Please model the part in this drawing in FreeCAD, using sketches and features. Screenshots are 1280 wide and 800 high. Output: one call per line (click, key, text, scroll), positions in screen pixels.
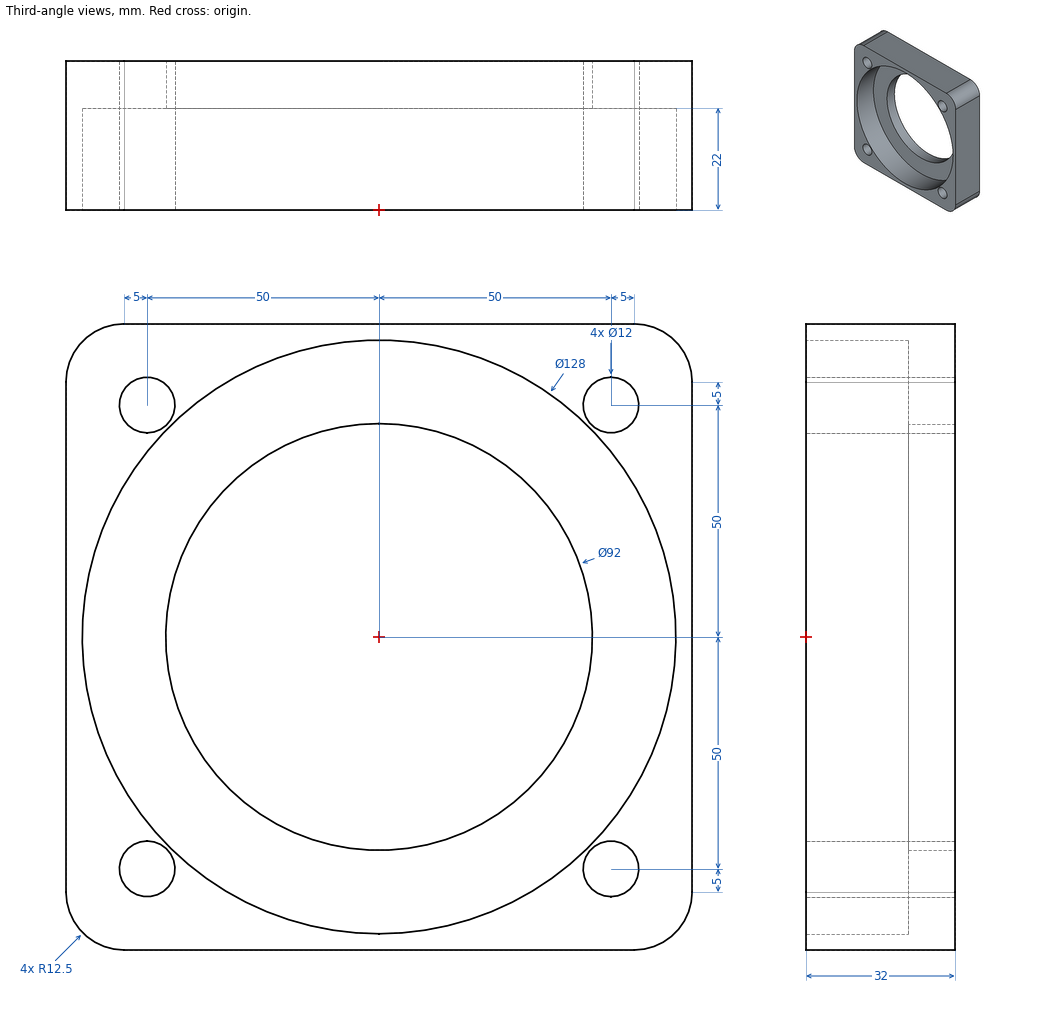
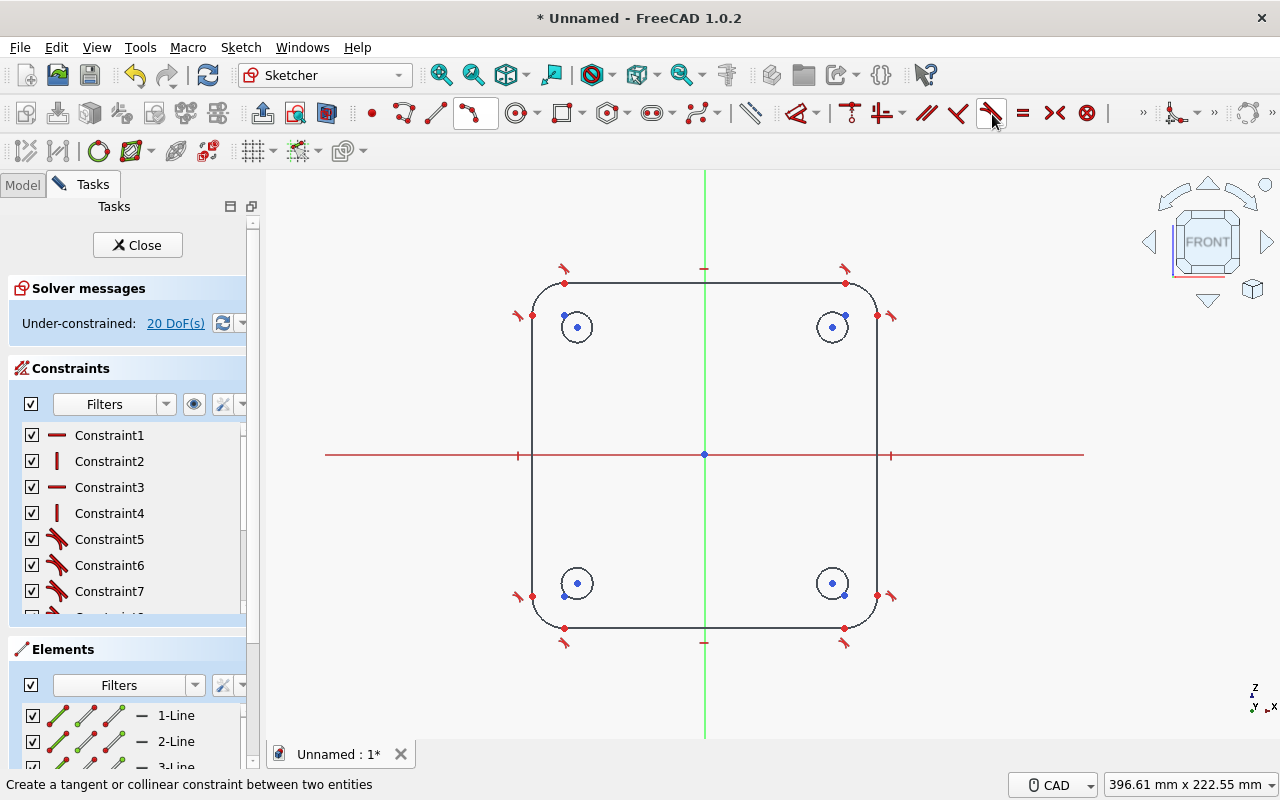
click(536, 611)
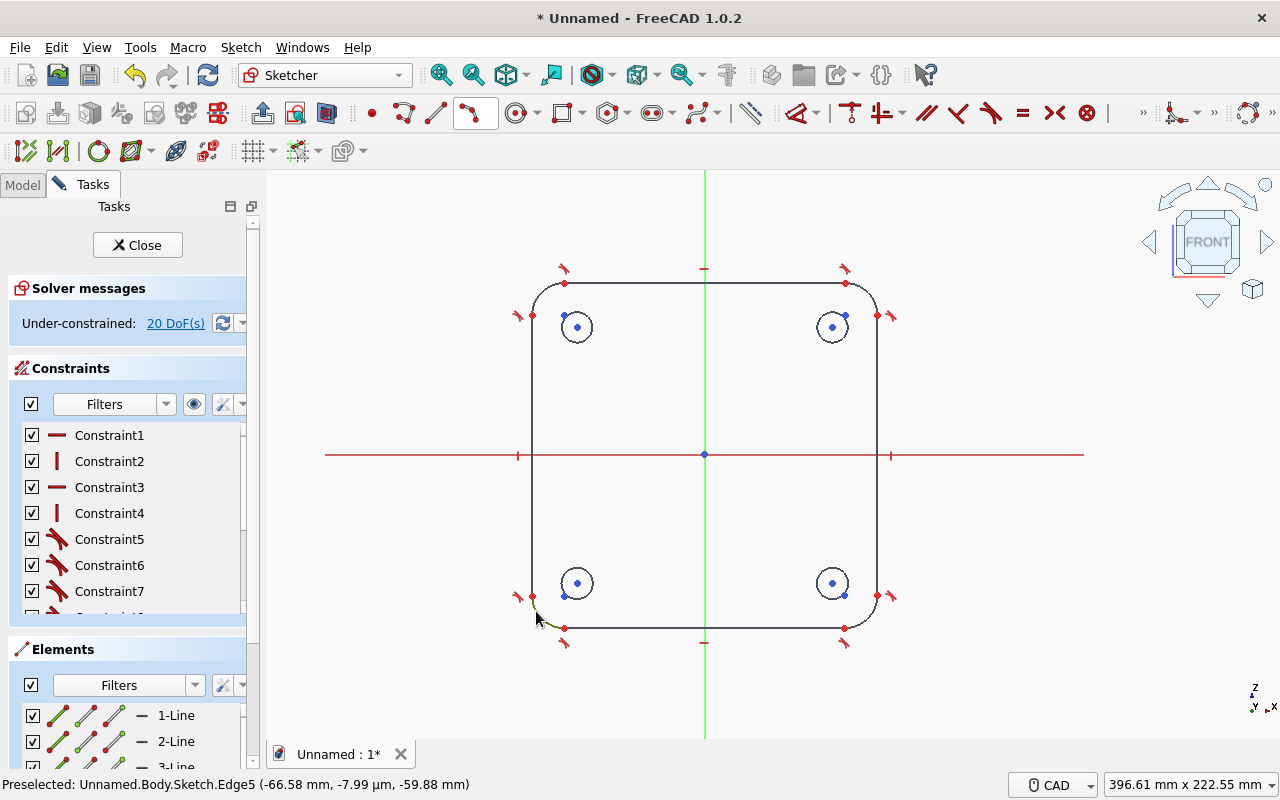
click(550, 287)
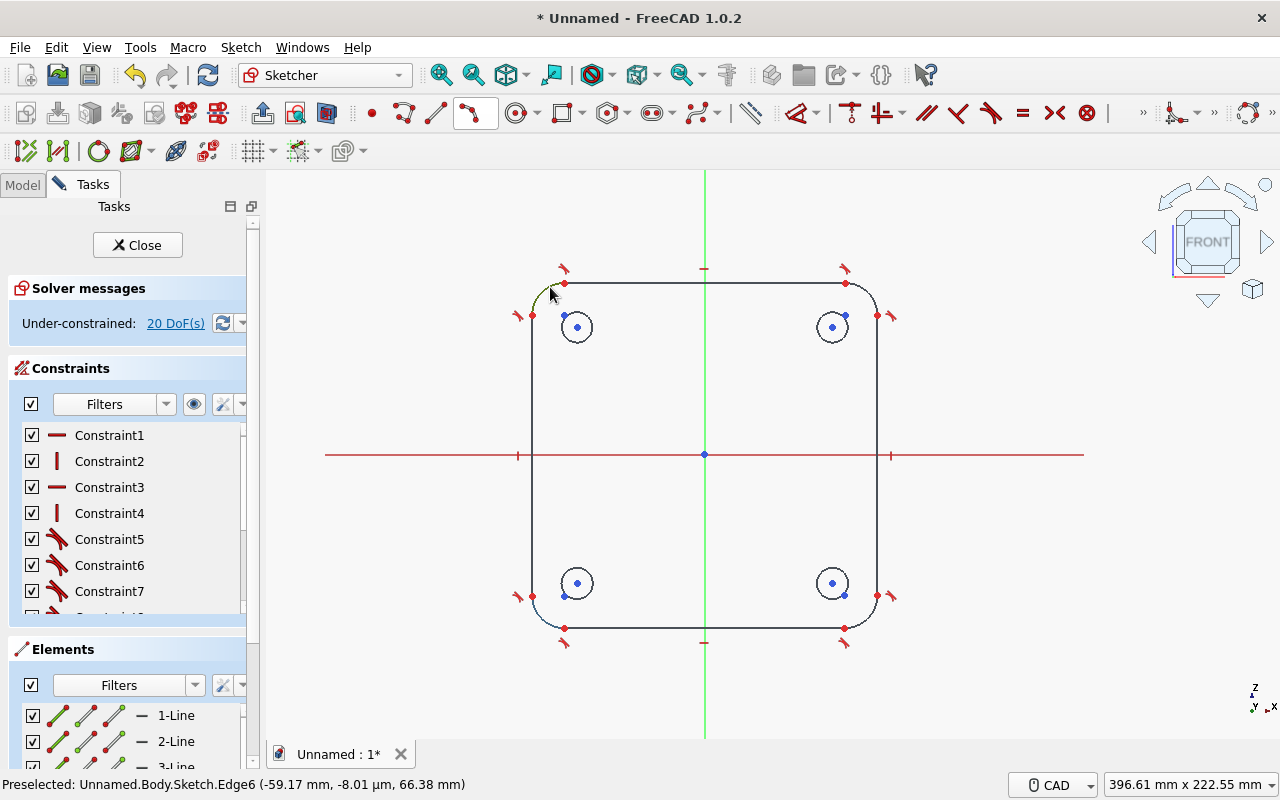
click(874, 301)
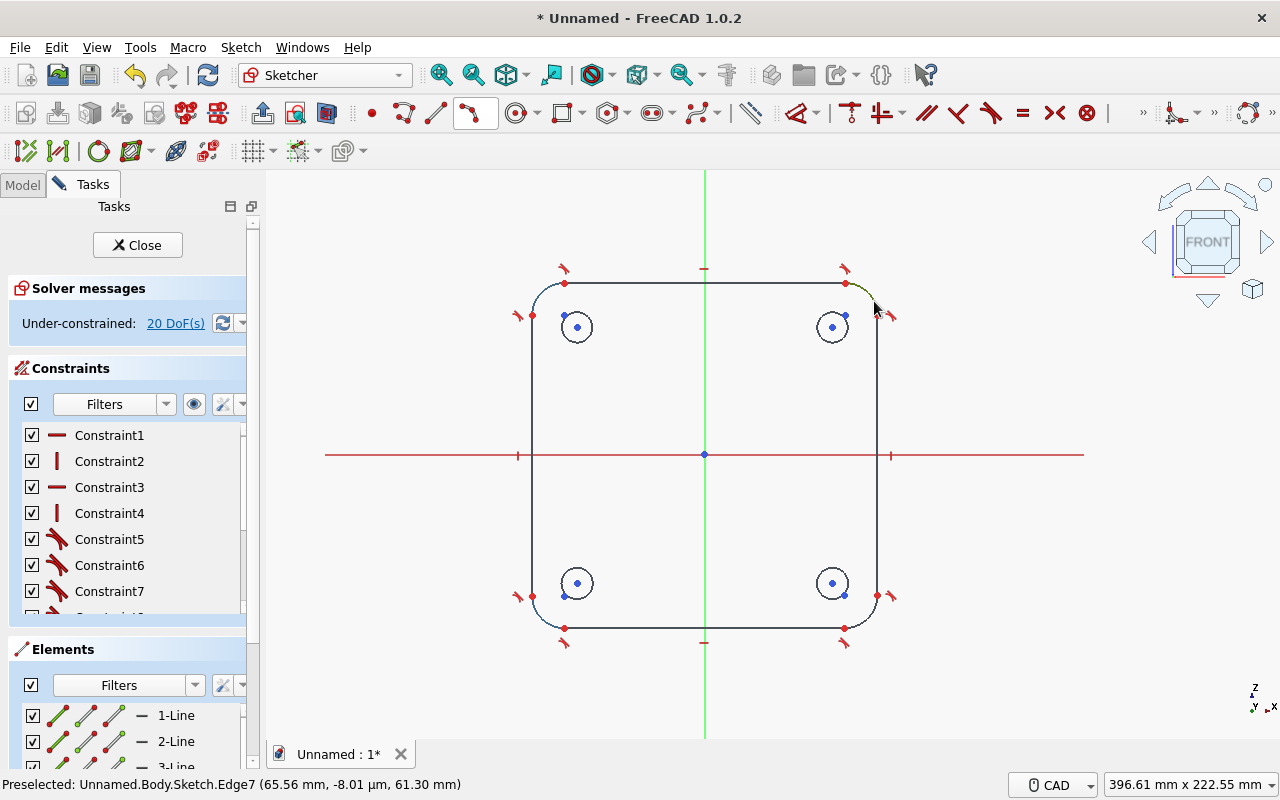
click(860, 625)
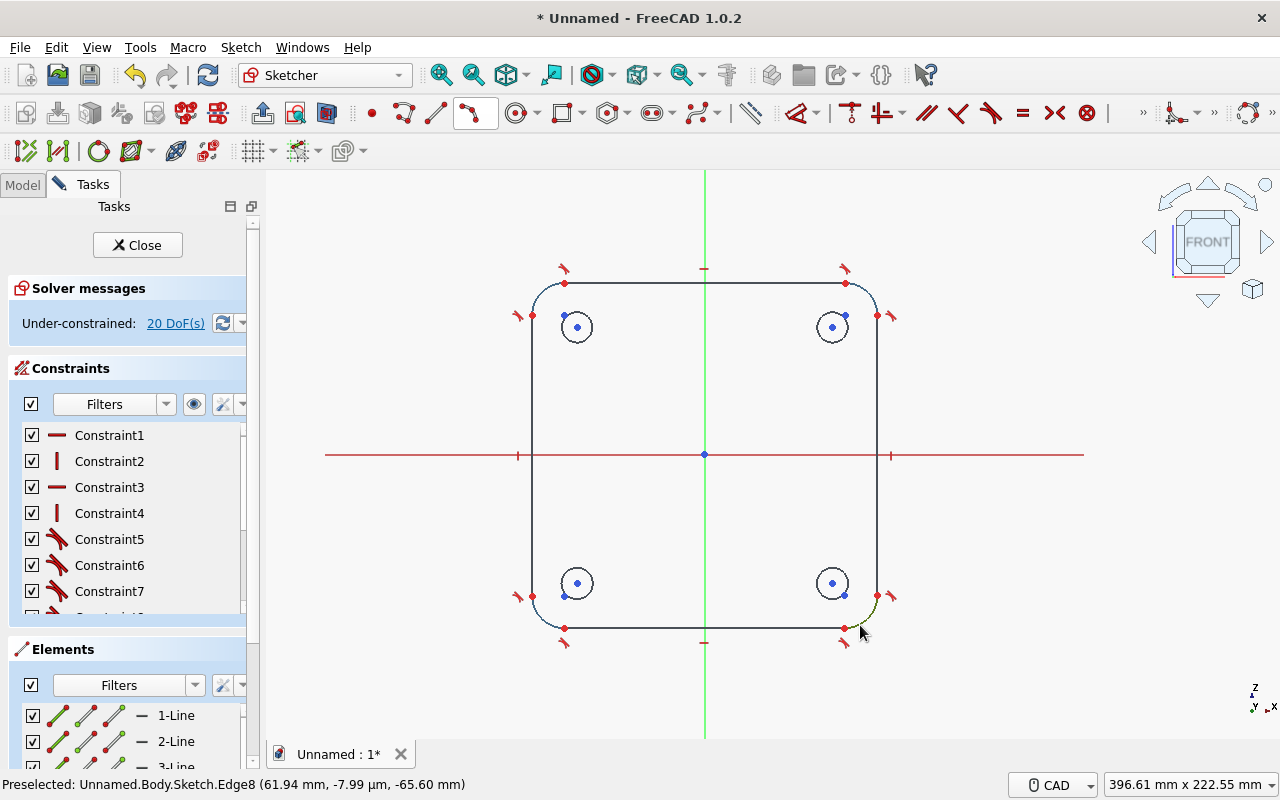
click(1024, 114)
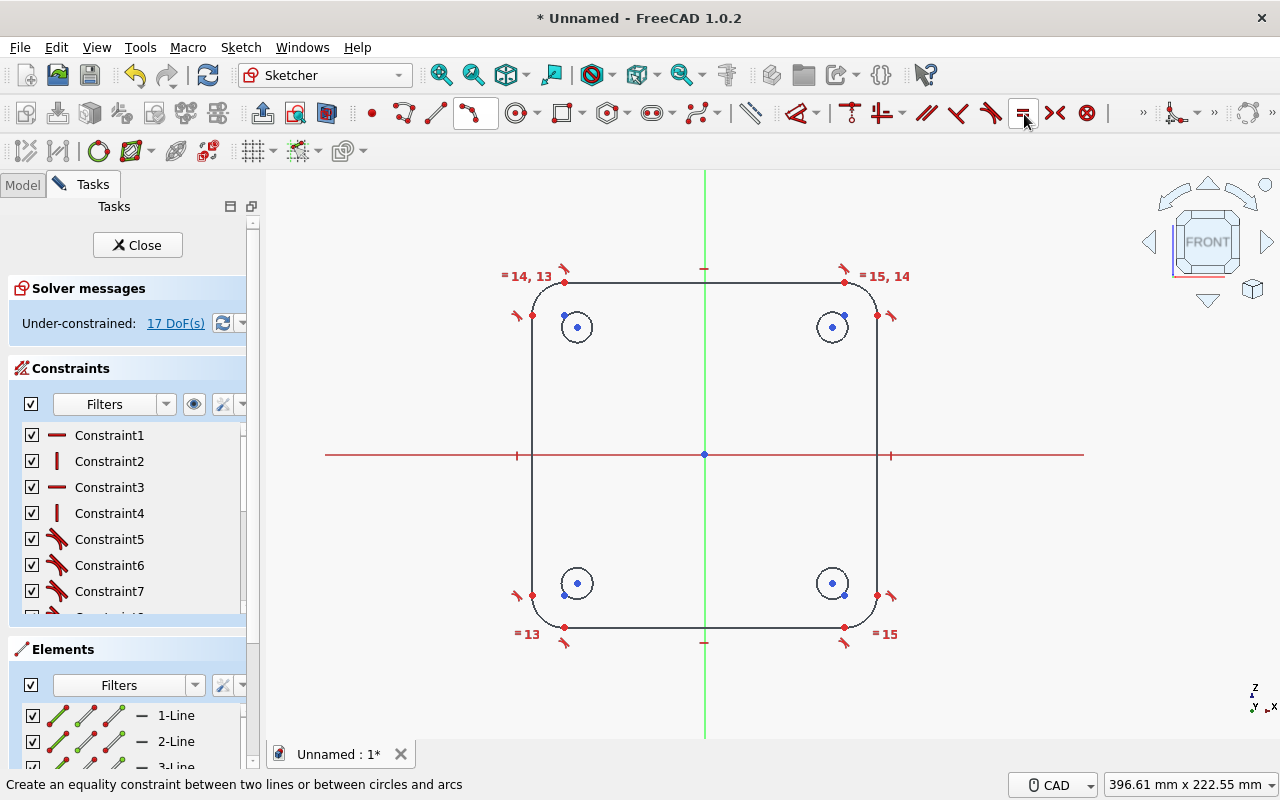
click(822, 317)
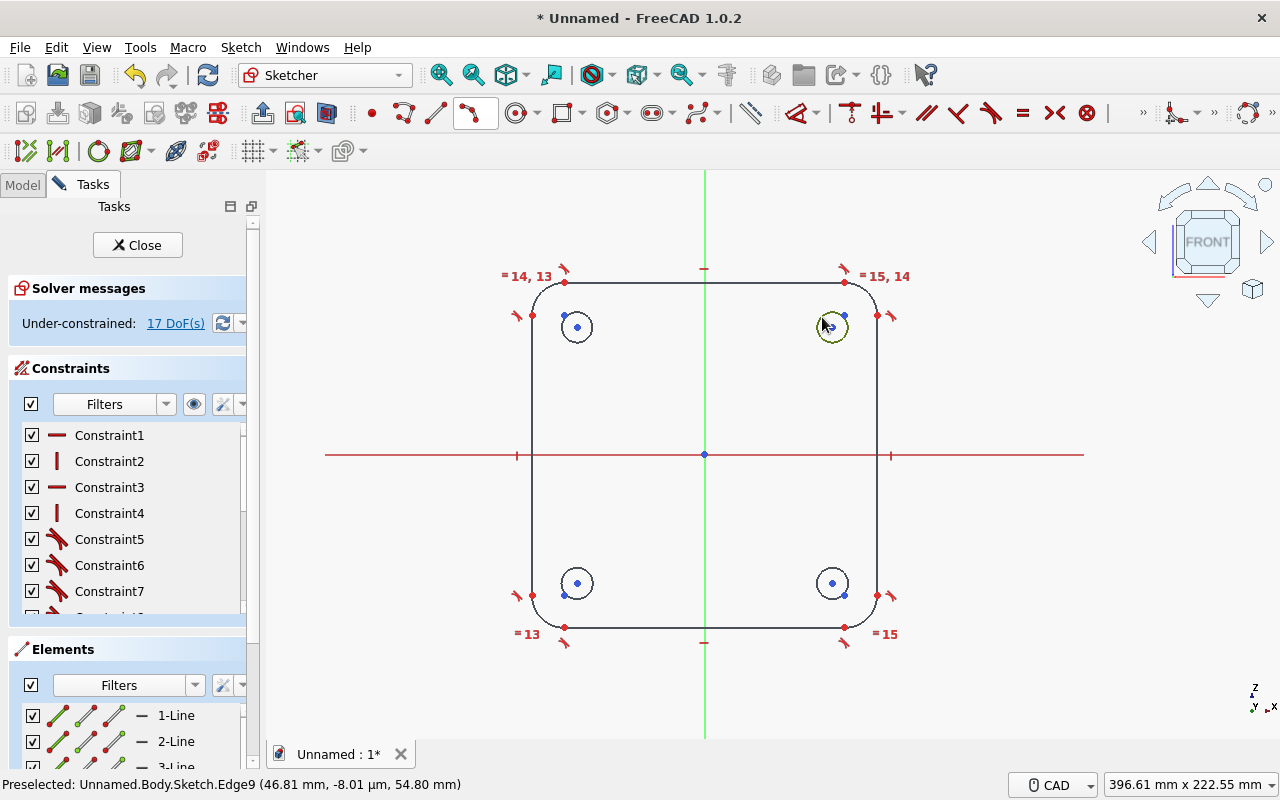
click(588, 317)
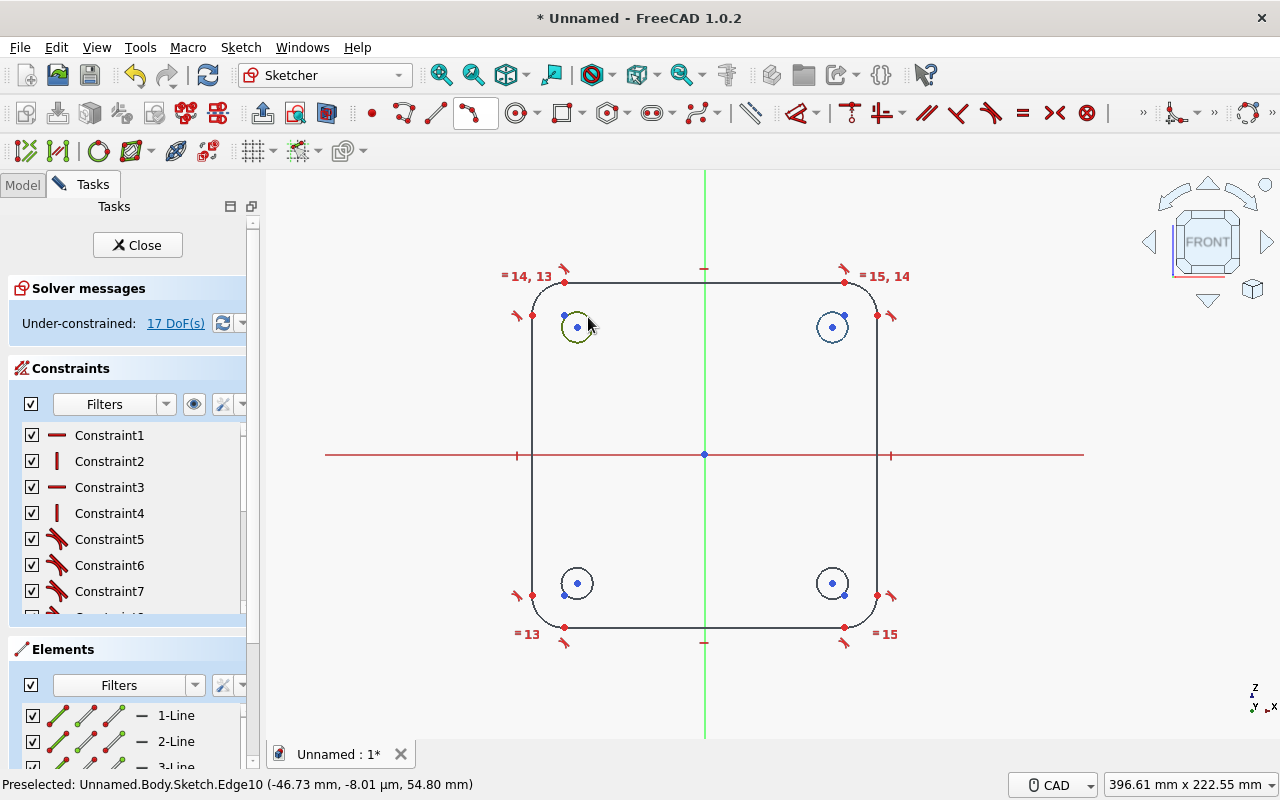
click(844, 572)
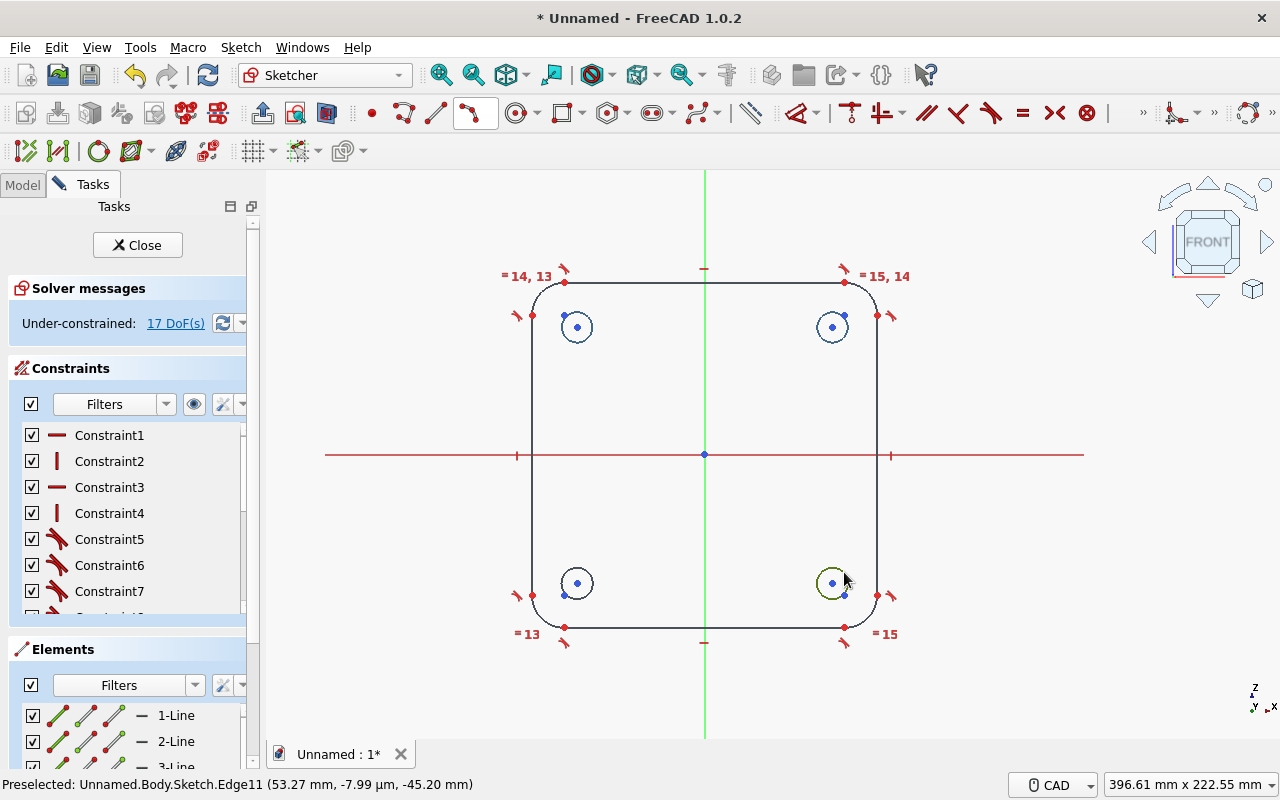
click(588, 572)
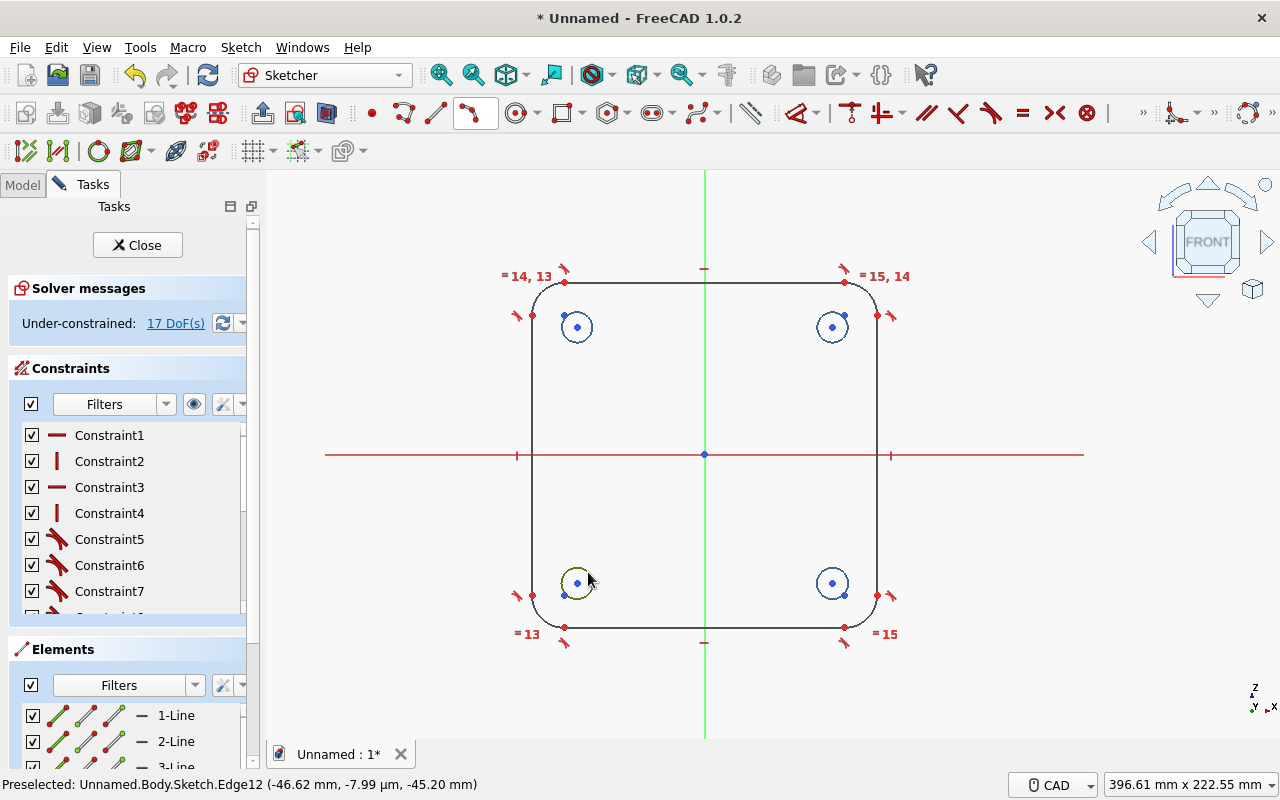
key(e)